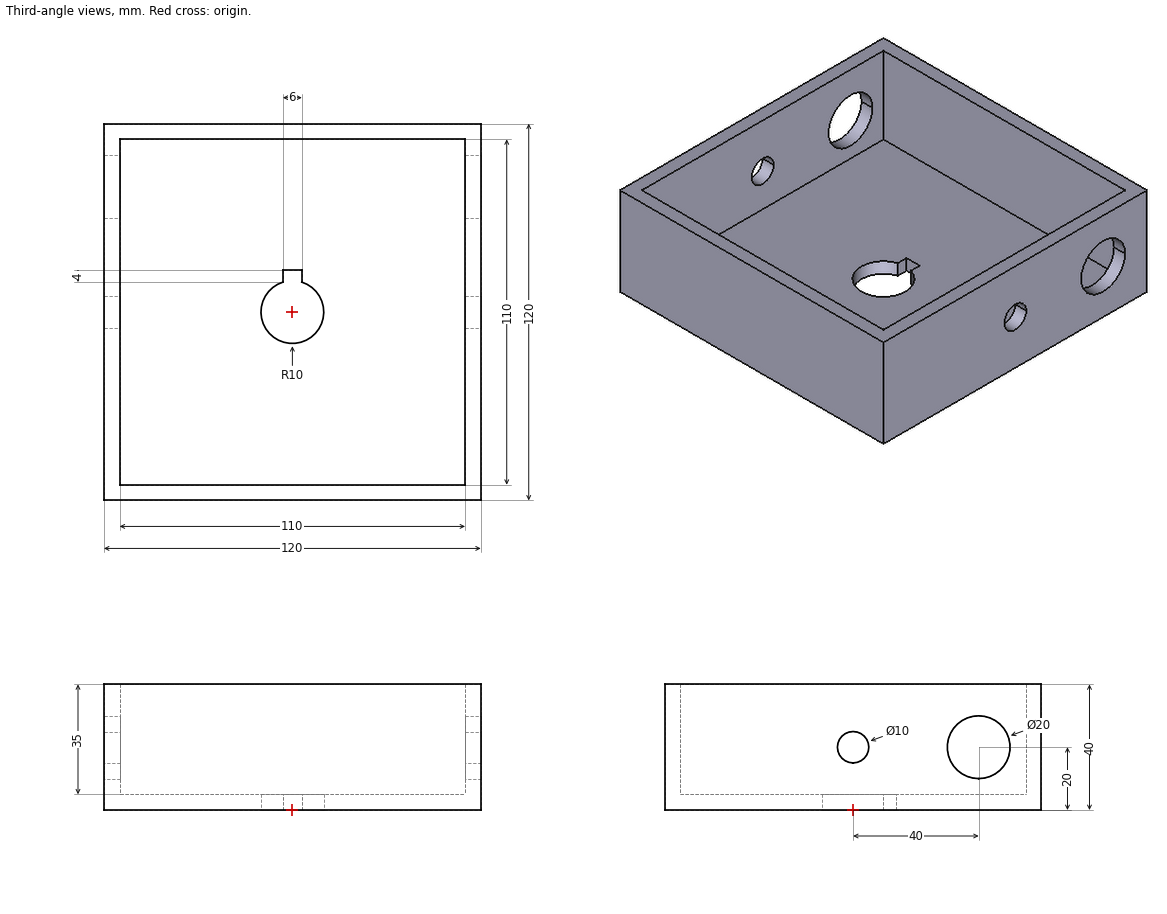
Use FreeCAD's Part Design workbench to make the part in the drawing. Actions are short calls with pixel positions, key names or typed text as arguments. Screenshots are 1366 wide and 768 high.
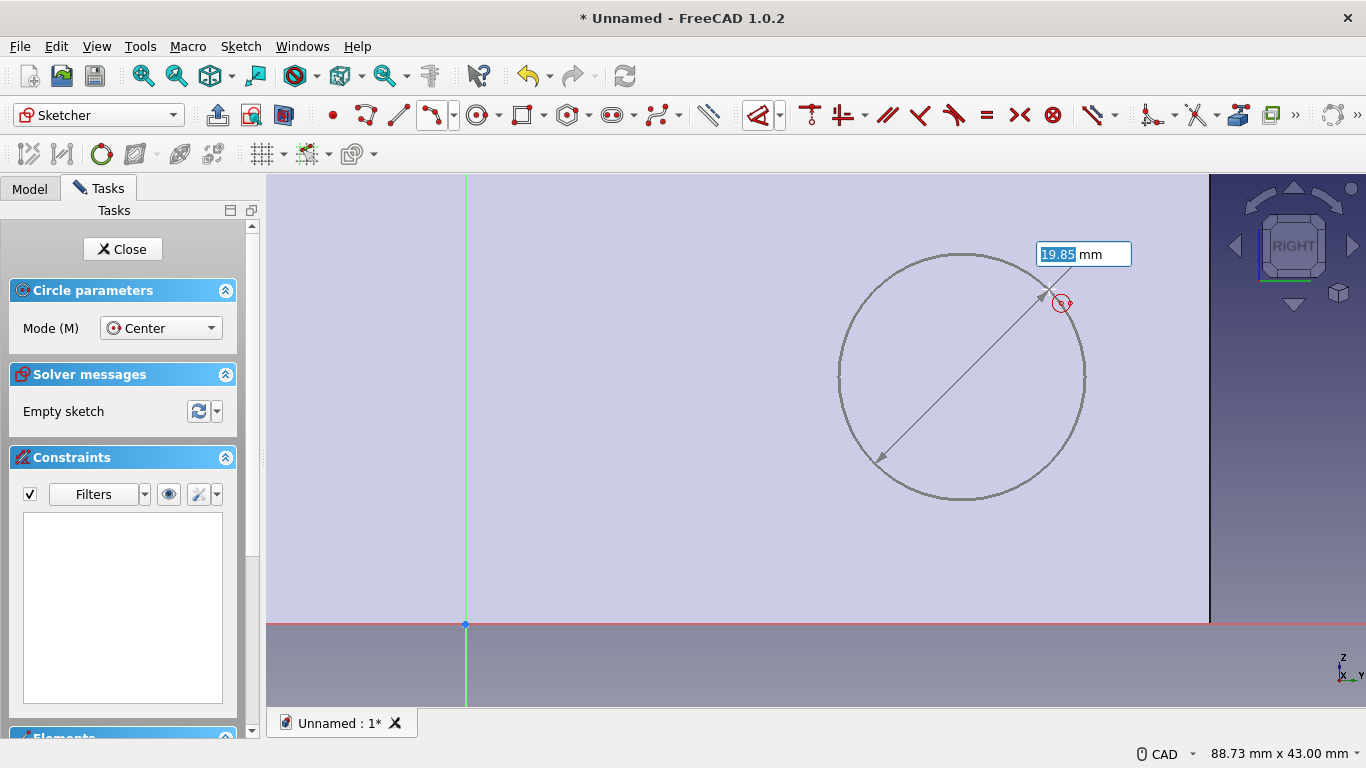
text(20)
key(Return)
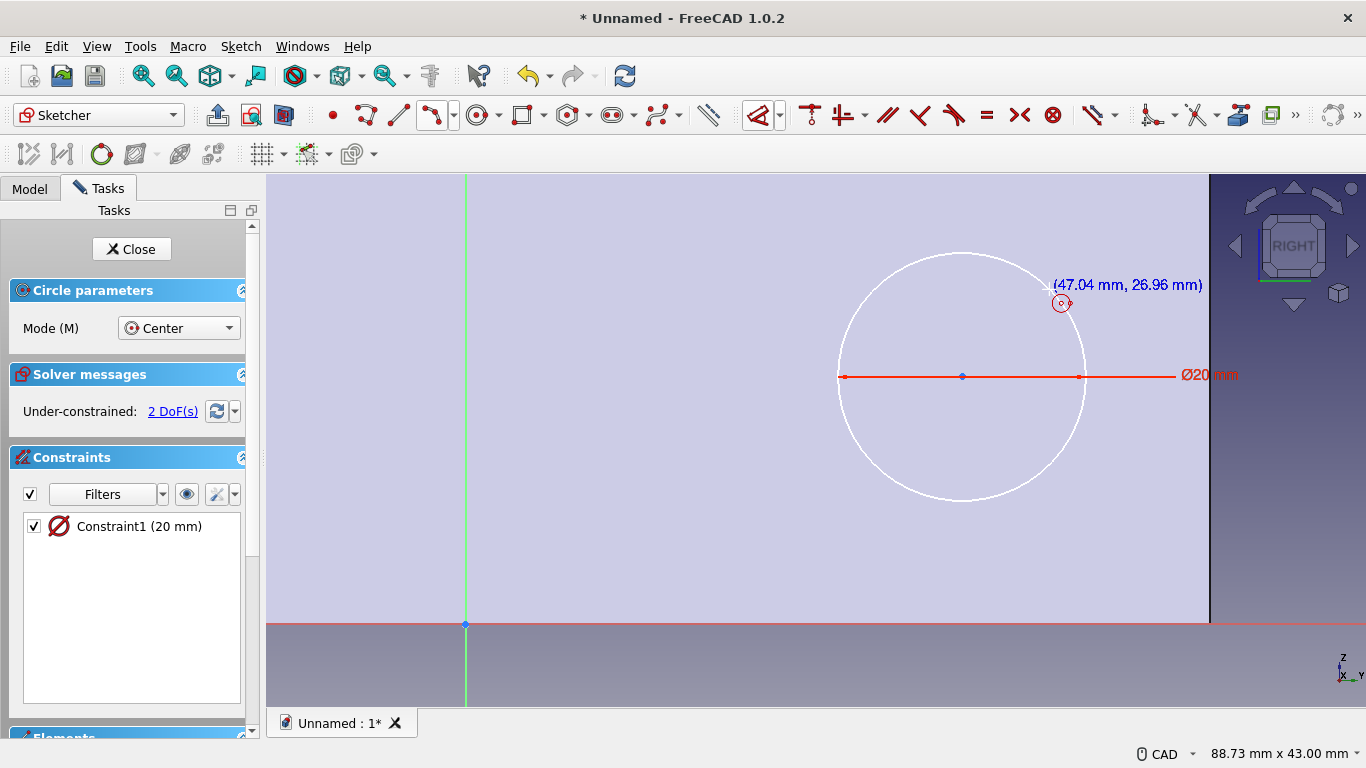
click(466, 376)
move(510, 332)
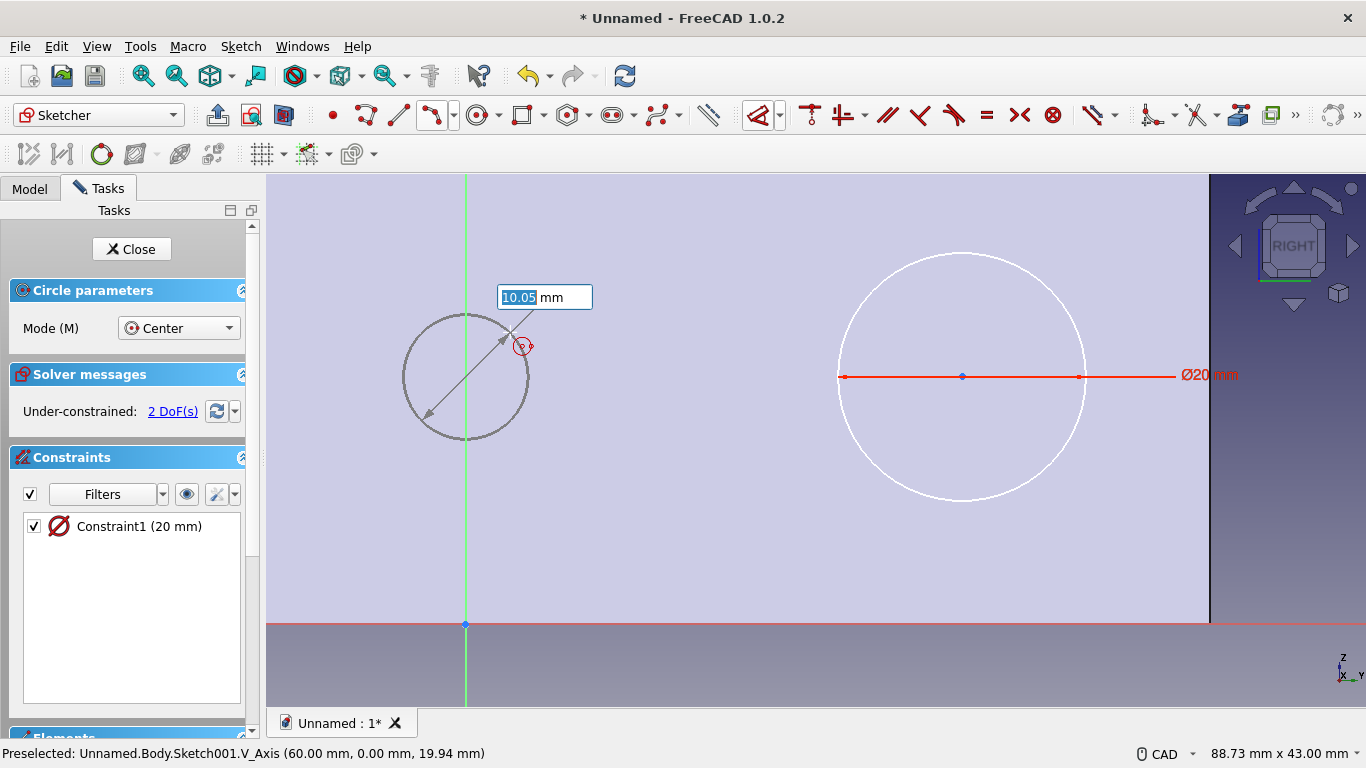
text(10)
key(Return)
key(Escape)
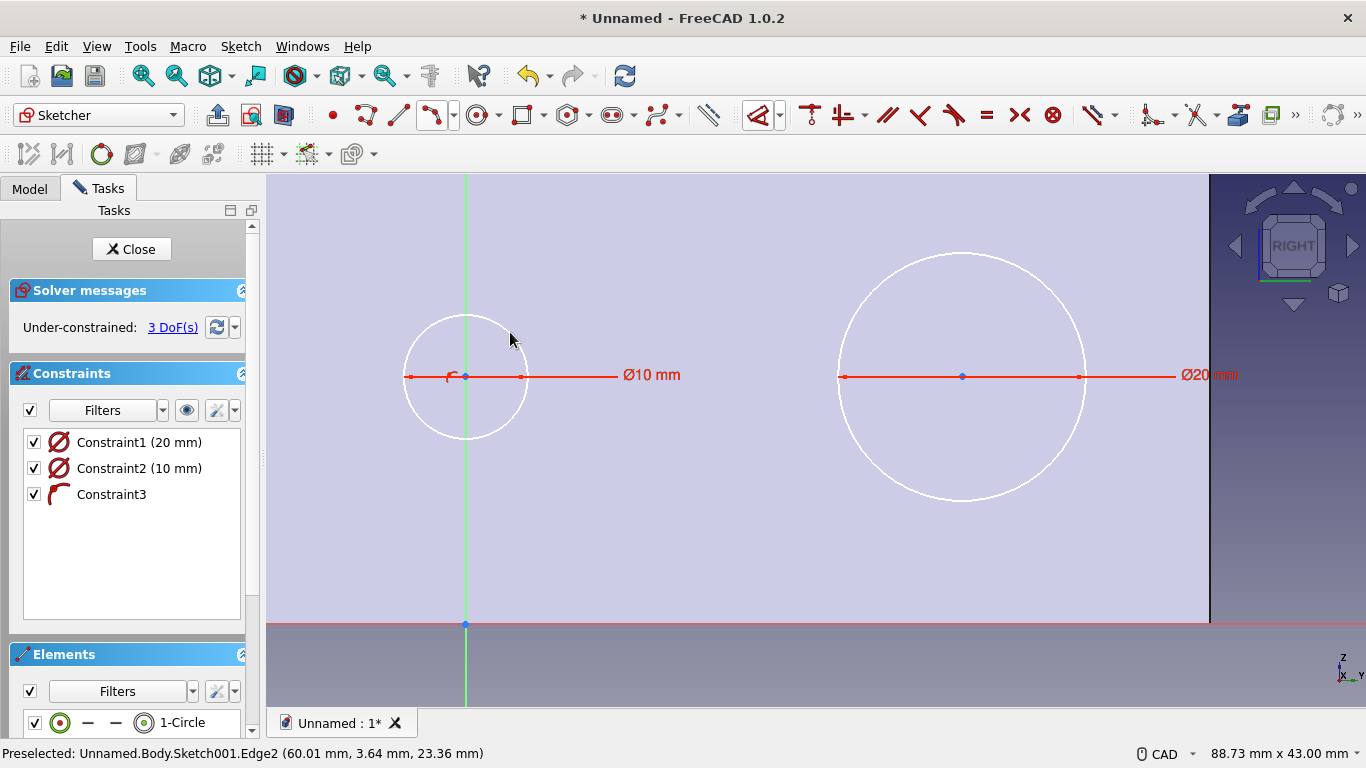
click(962, 377)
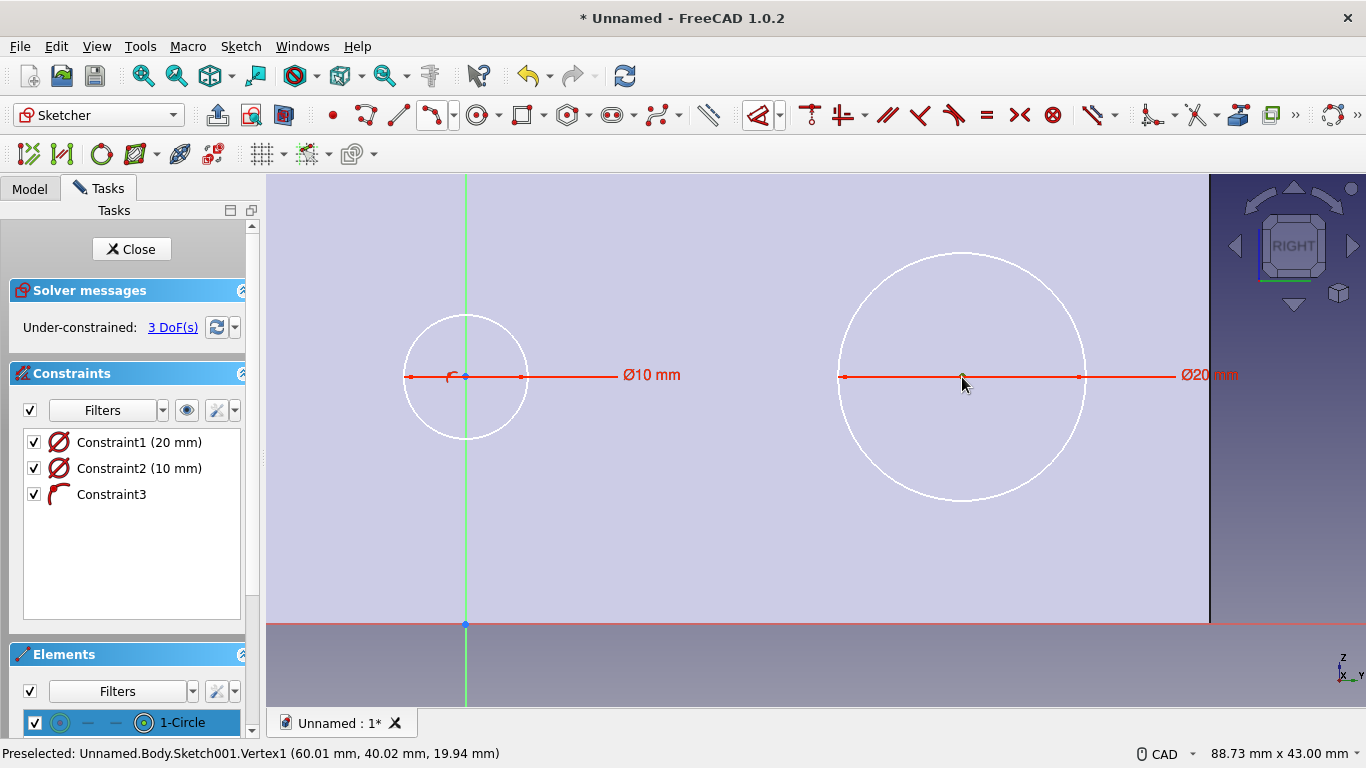
key(l)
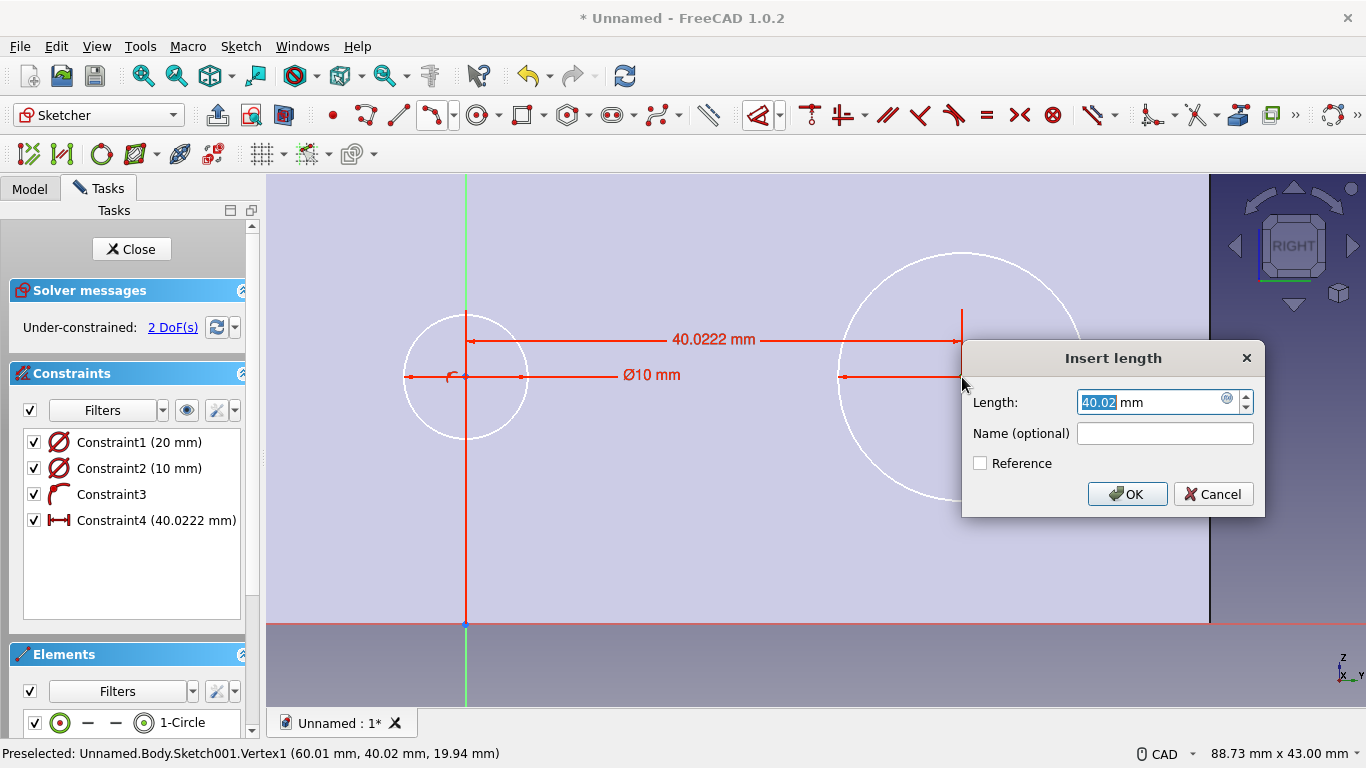
text(40)
key(Return)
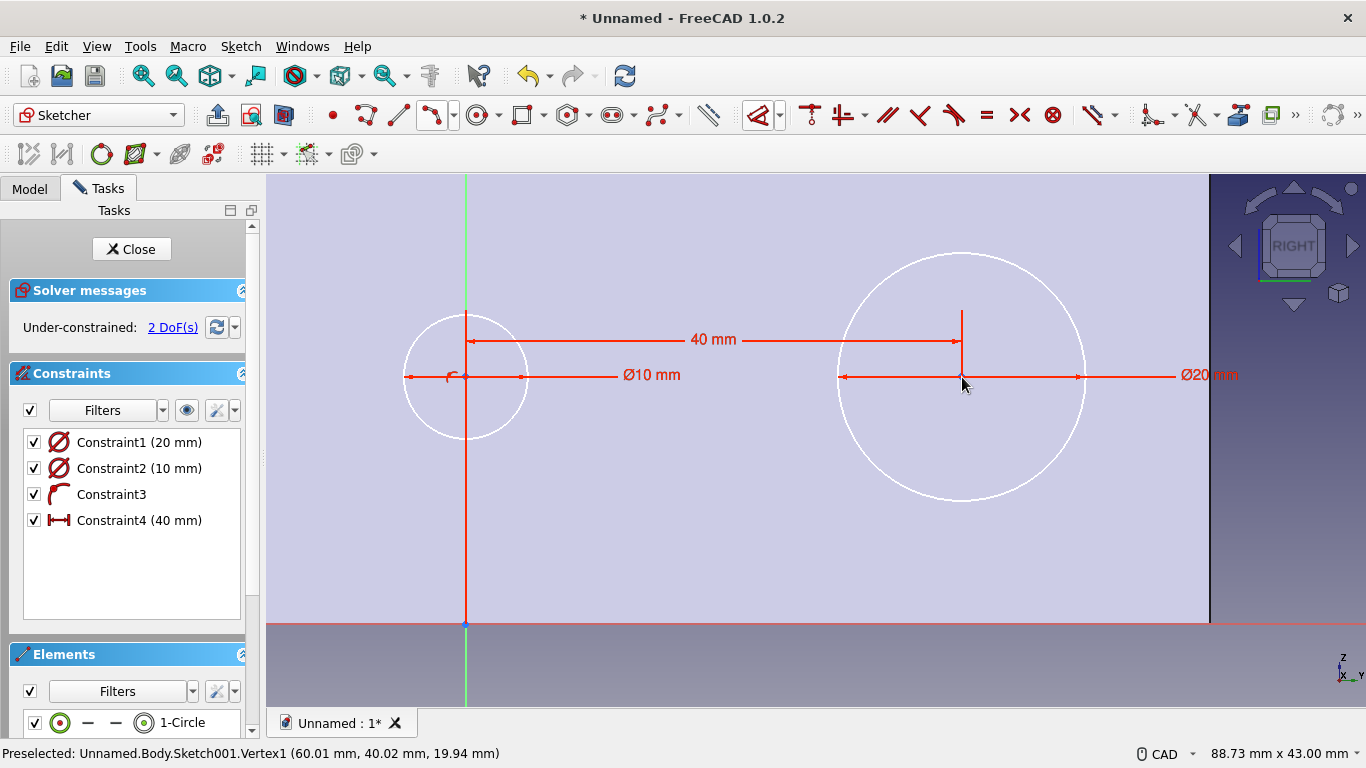
click(962, 377)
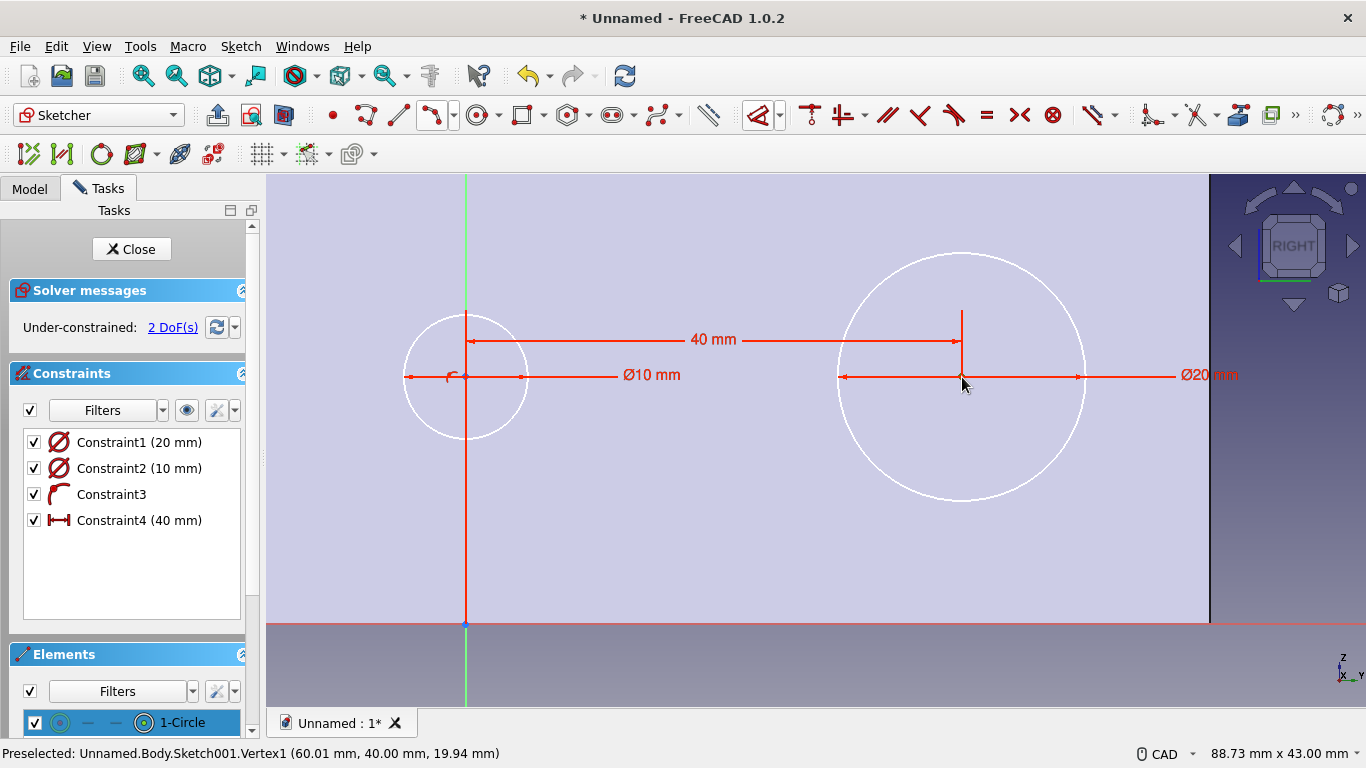
key(i)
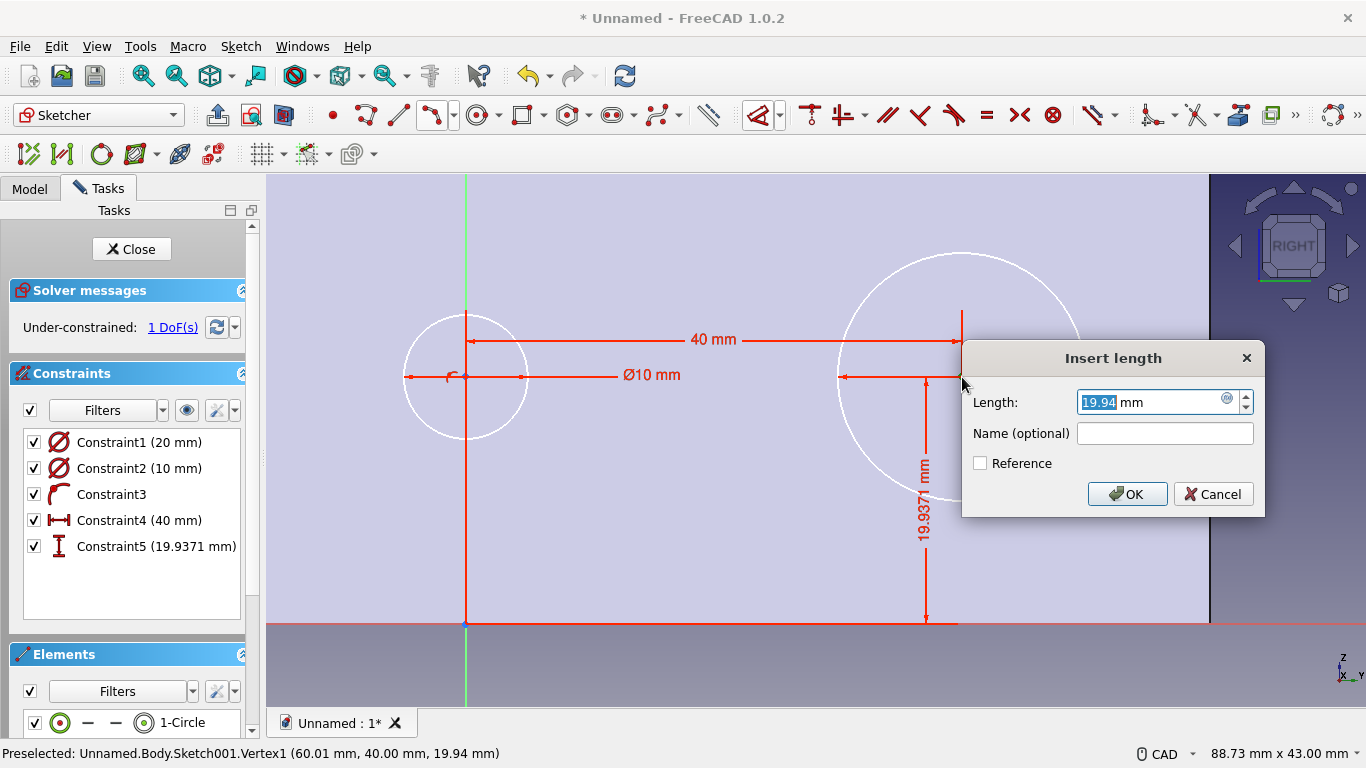
text(20)
key(Return)